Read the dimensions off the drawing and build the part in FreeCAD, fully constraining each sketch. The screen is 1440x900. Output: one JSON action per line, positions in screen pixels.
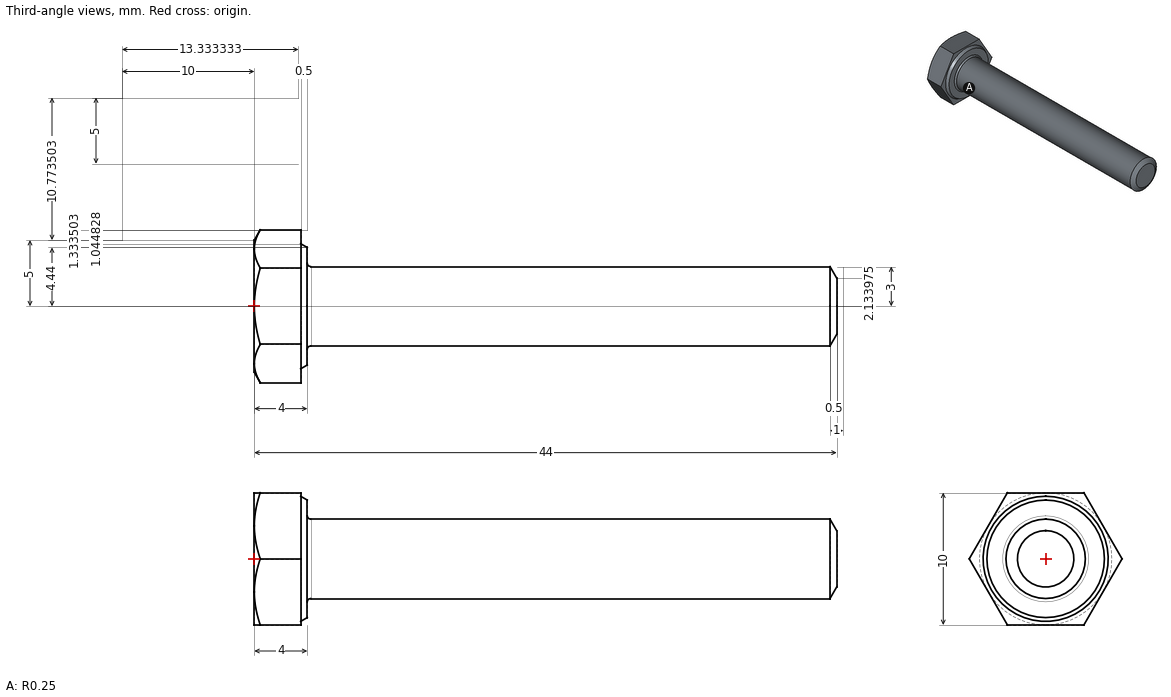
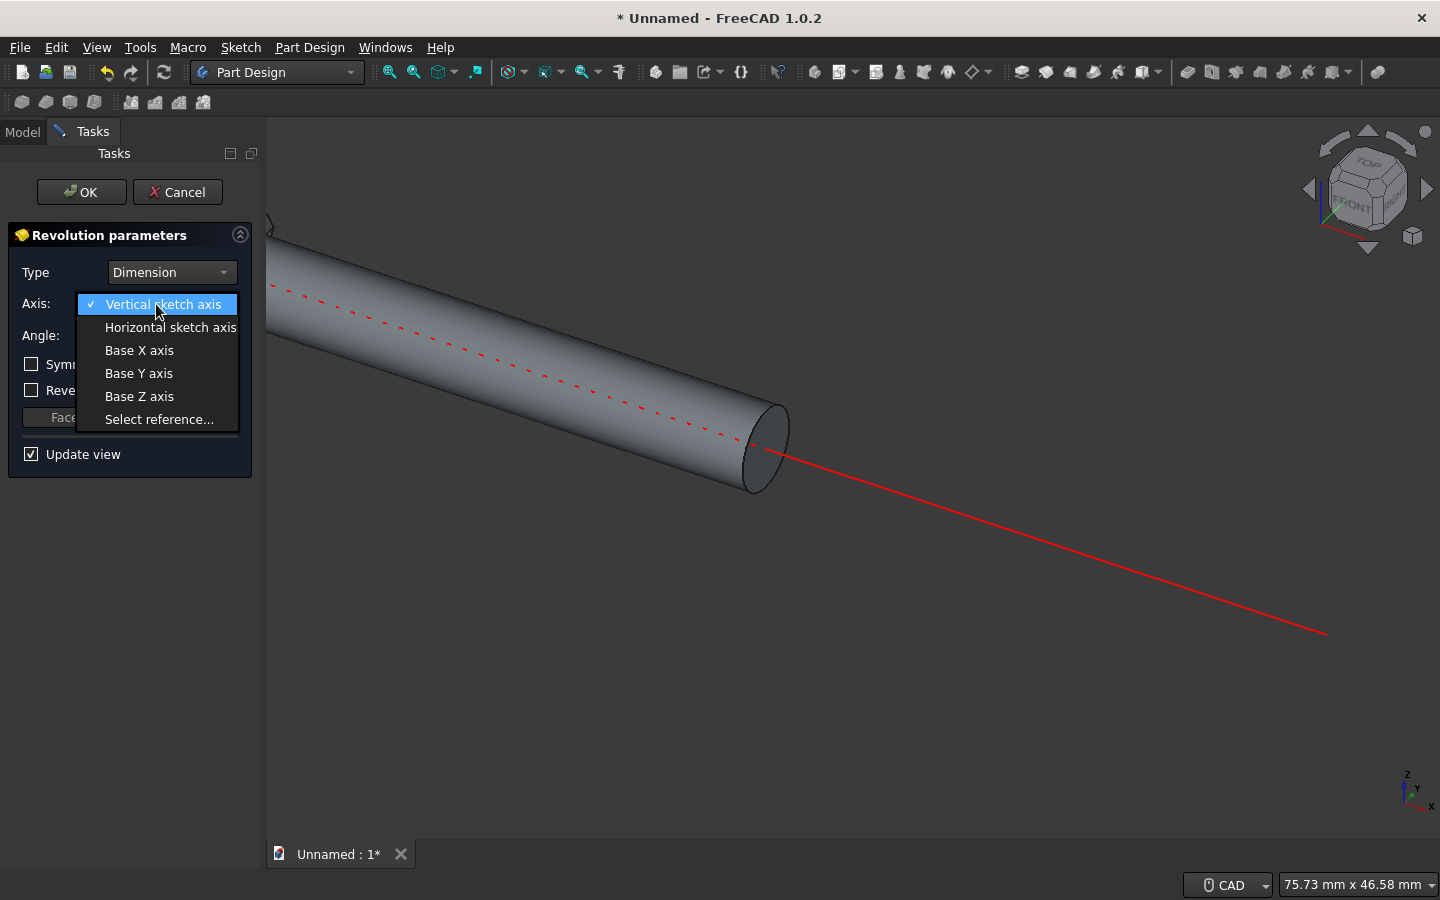
{"action": "left_click", "coordinate": [156, 328]}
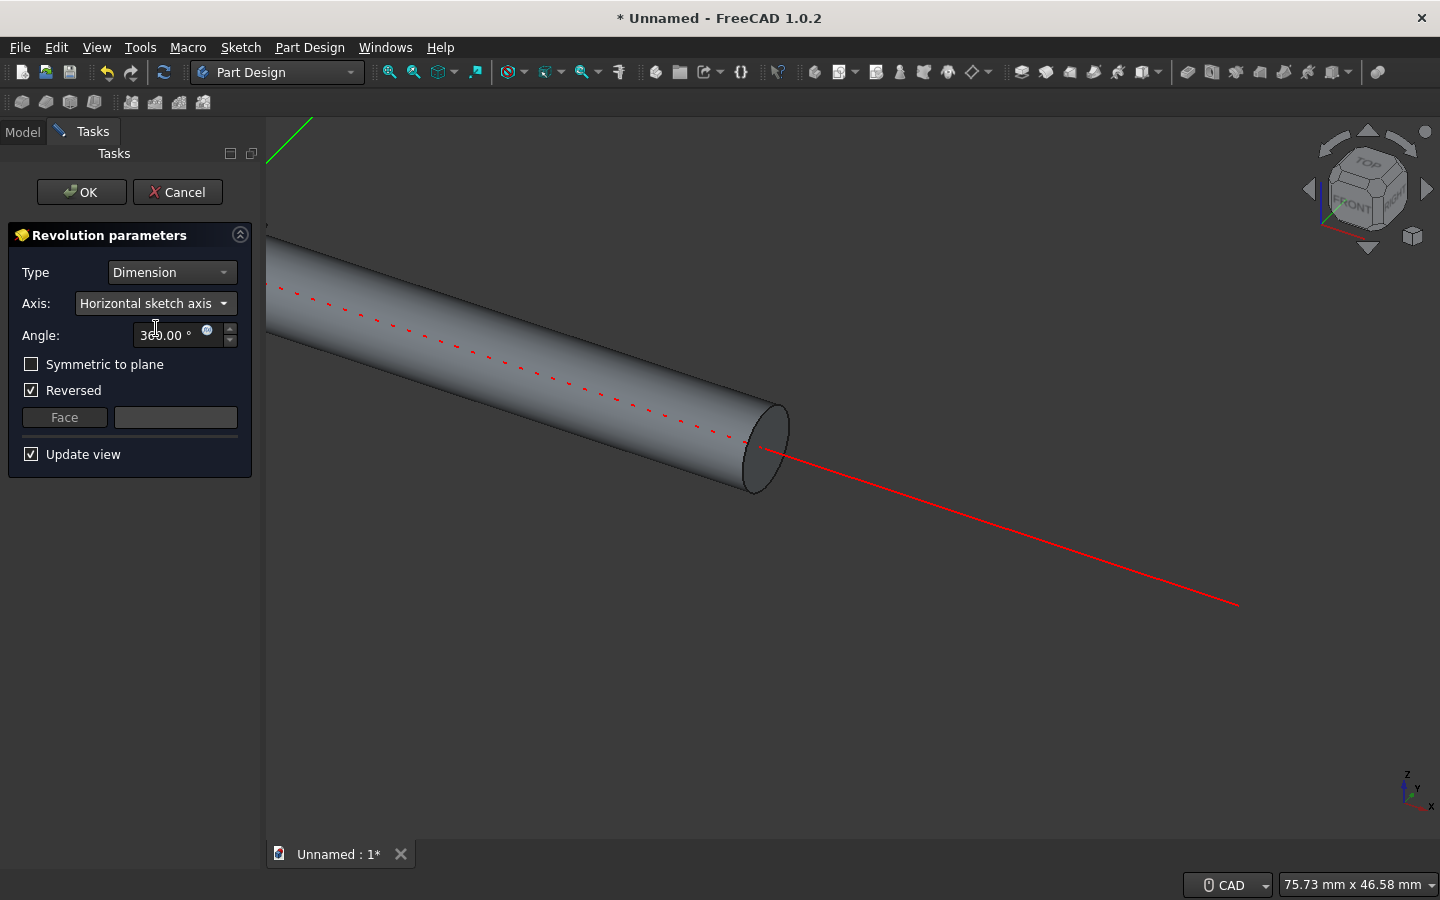
{"action": "left_click", "coordinate": [82, 192]}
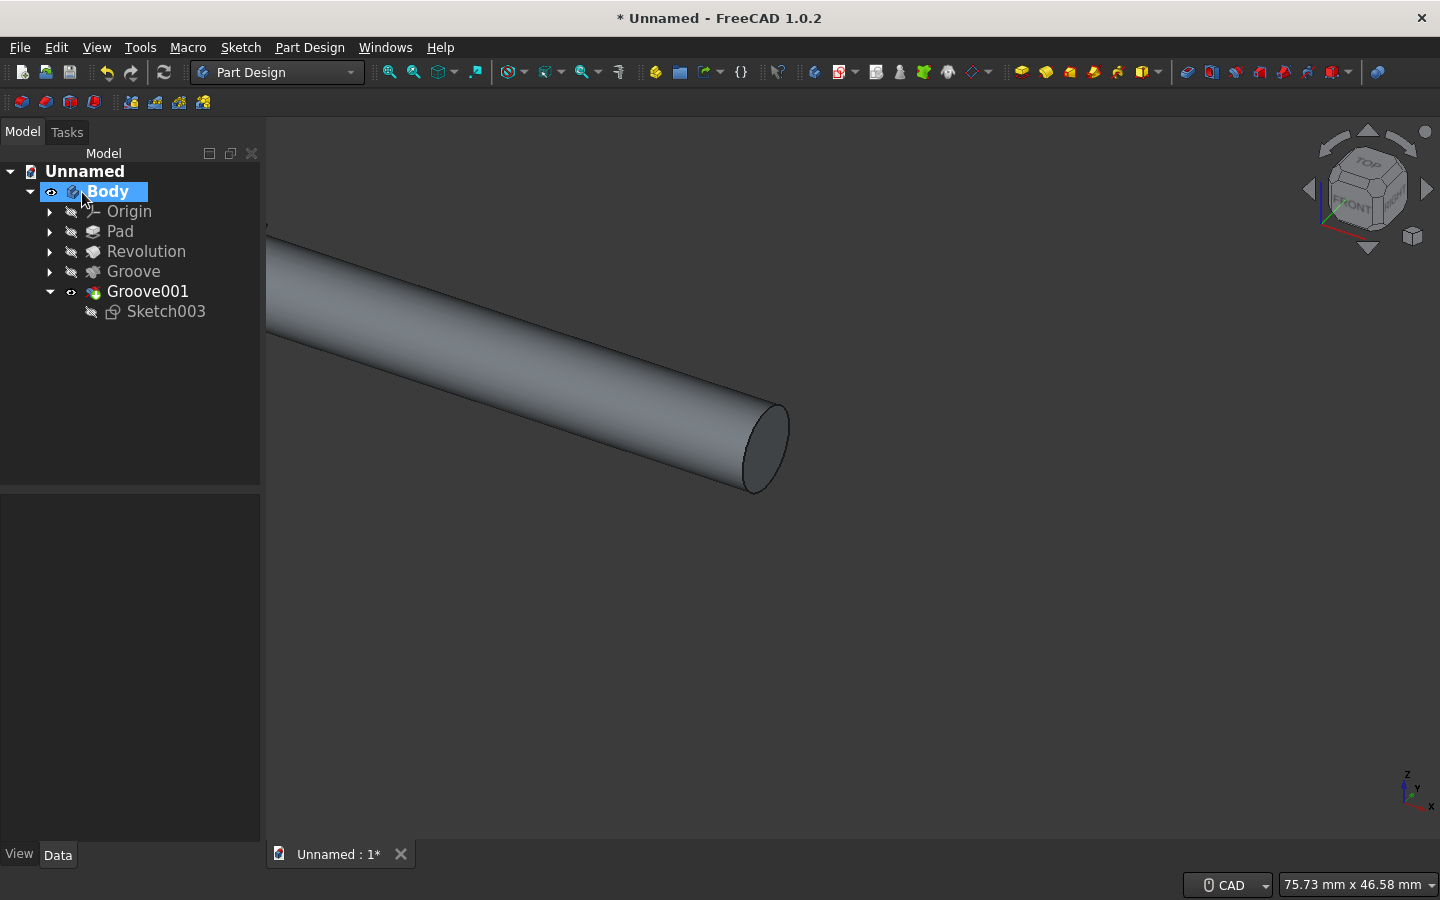
{"action": "left_click", "coordinate": [390, 72]}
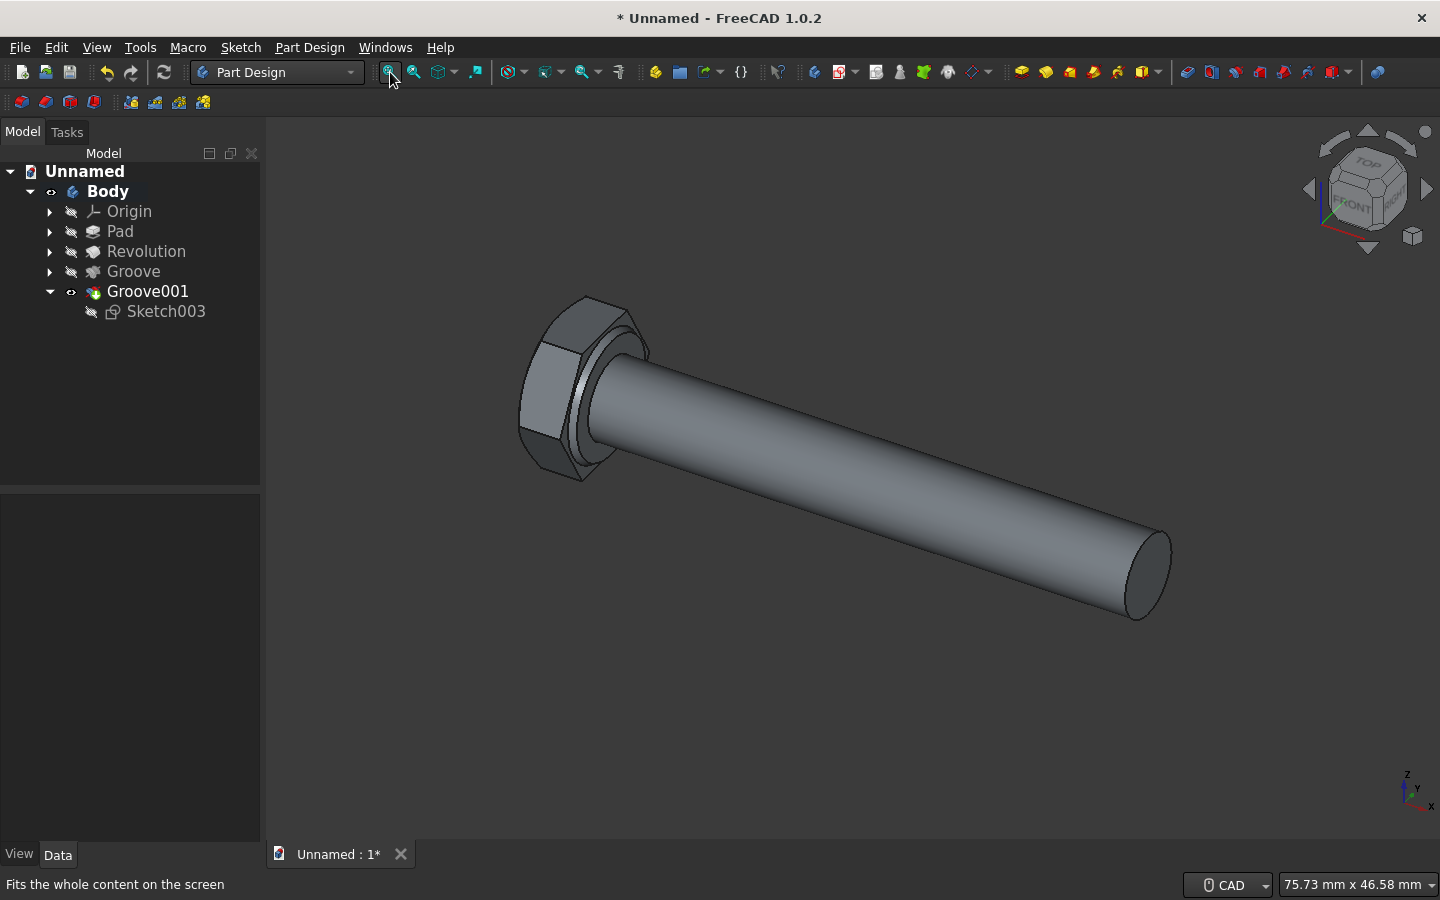
{"action": "key", "text": "0"}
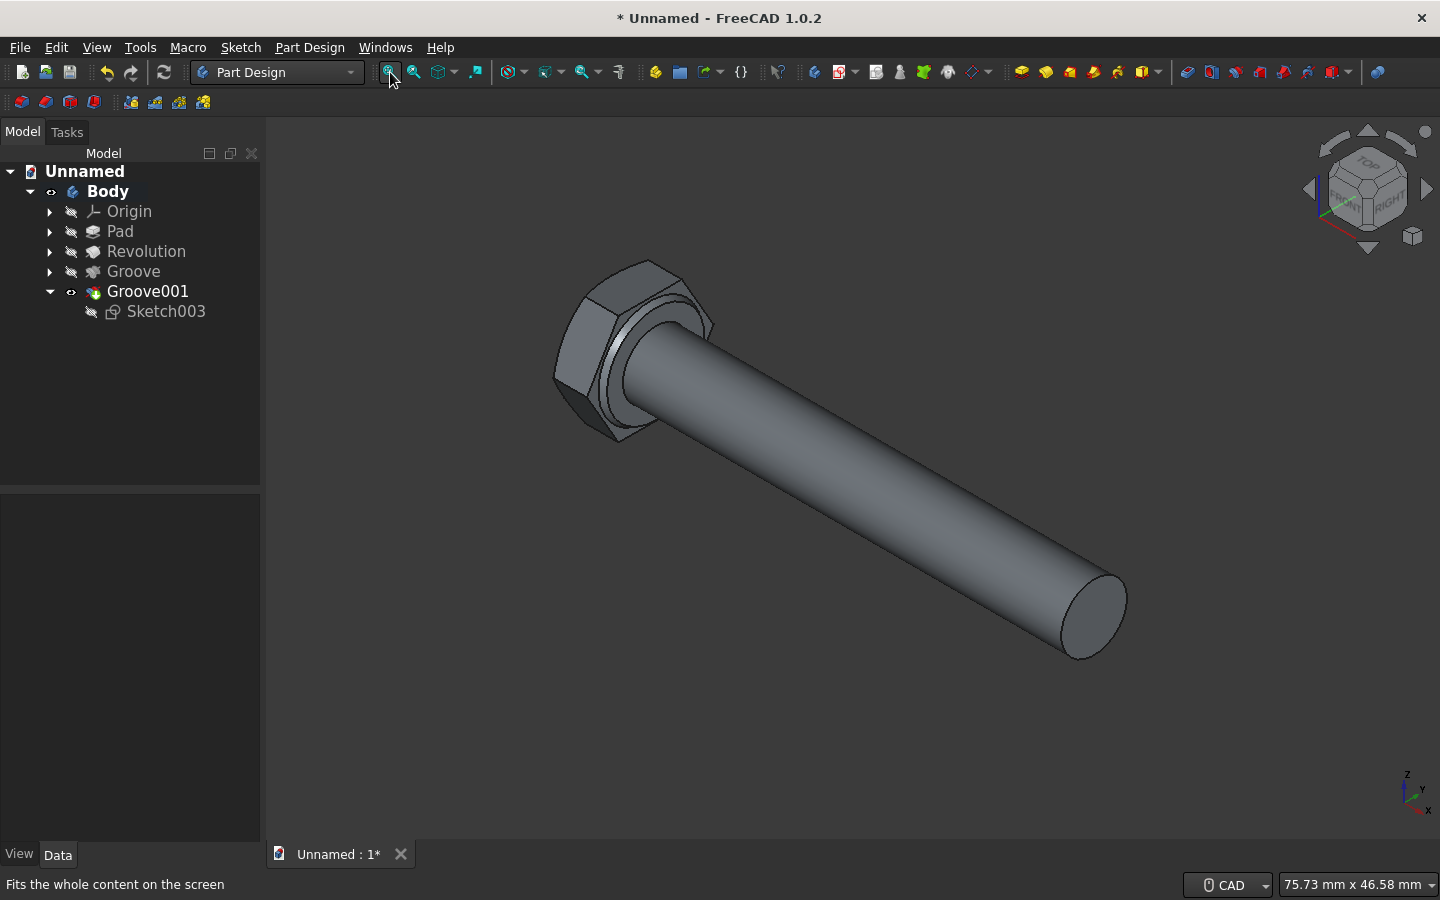
{"action": "key", "text": "2"}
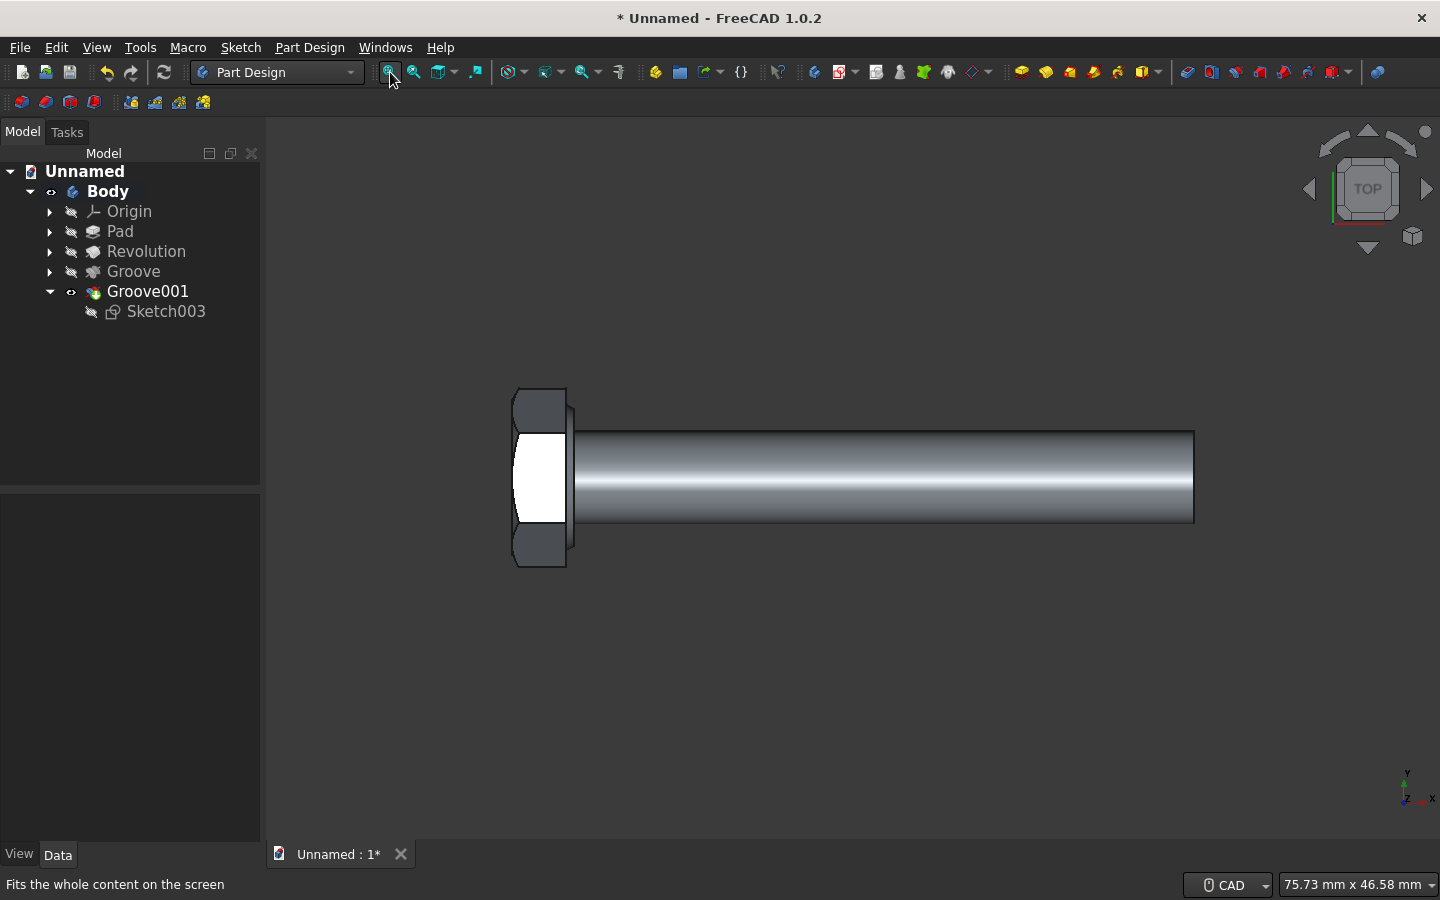
{"action": "key", "text": "1"}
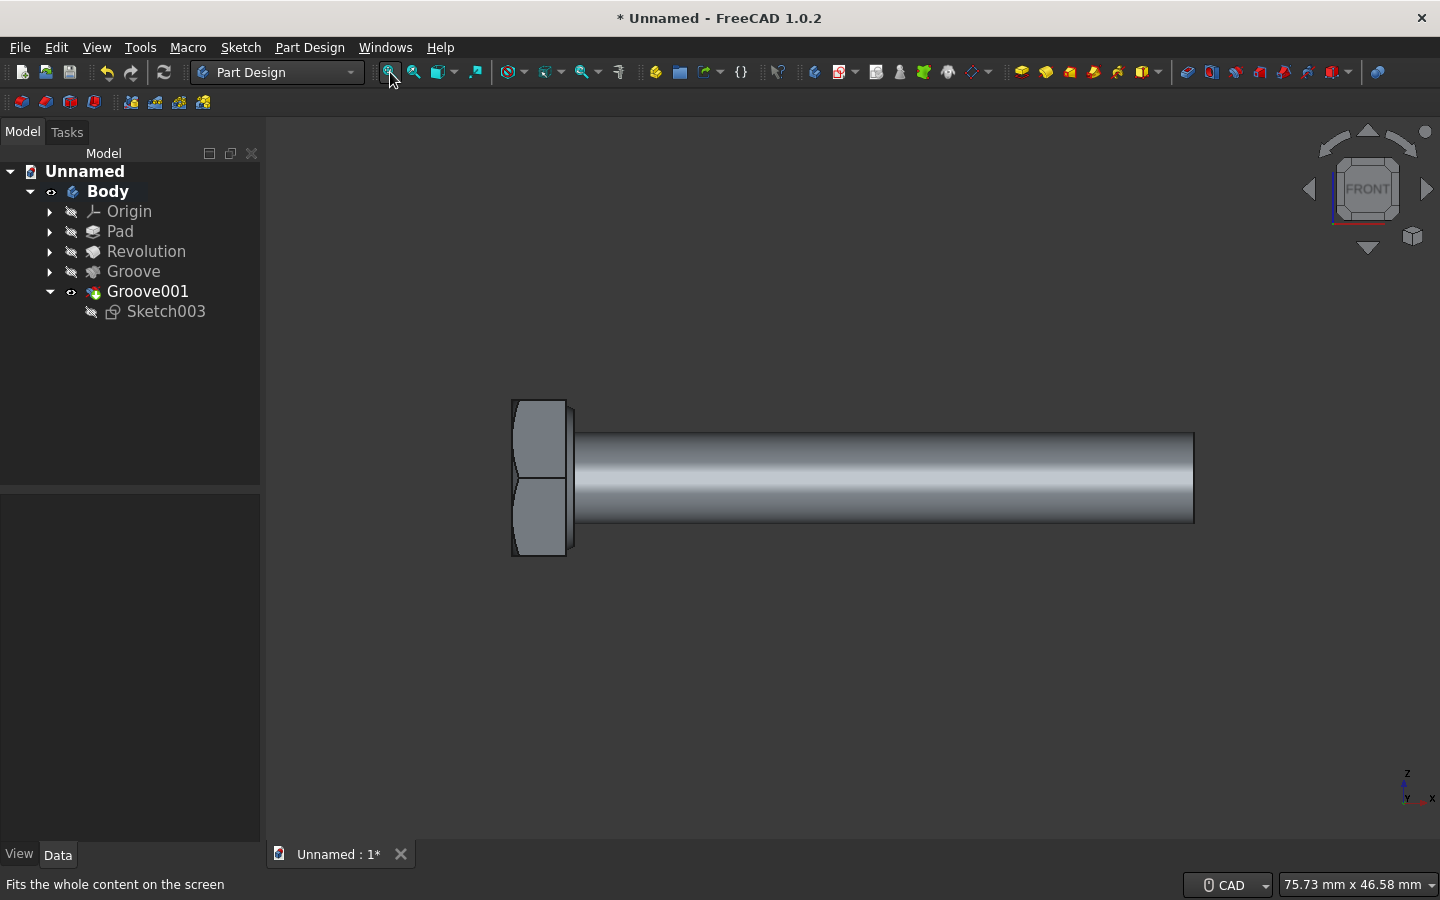
{"action": "key", "text": "3"}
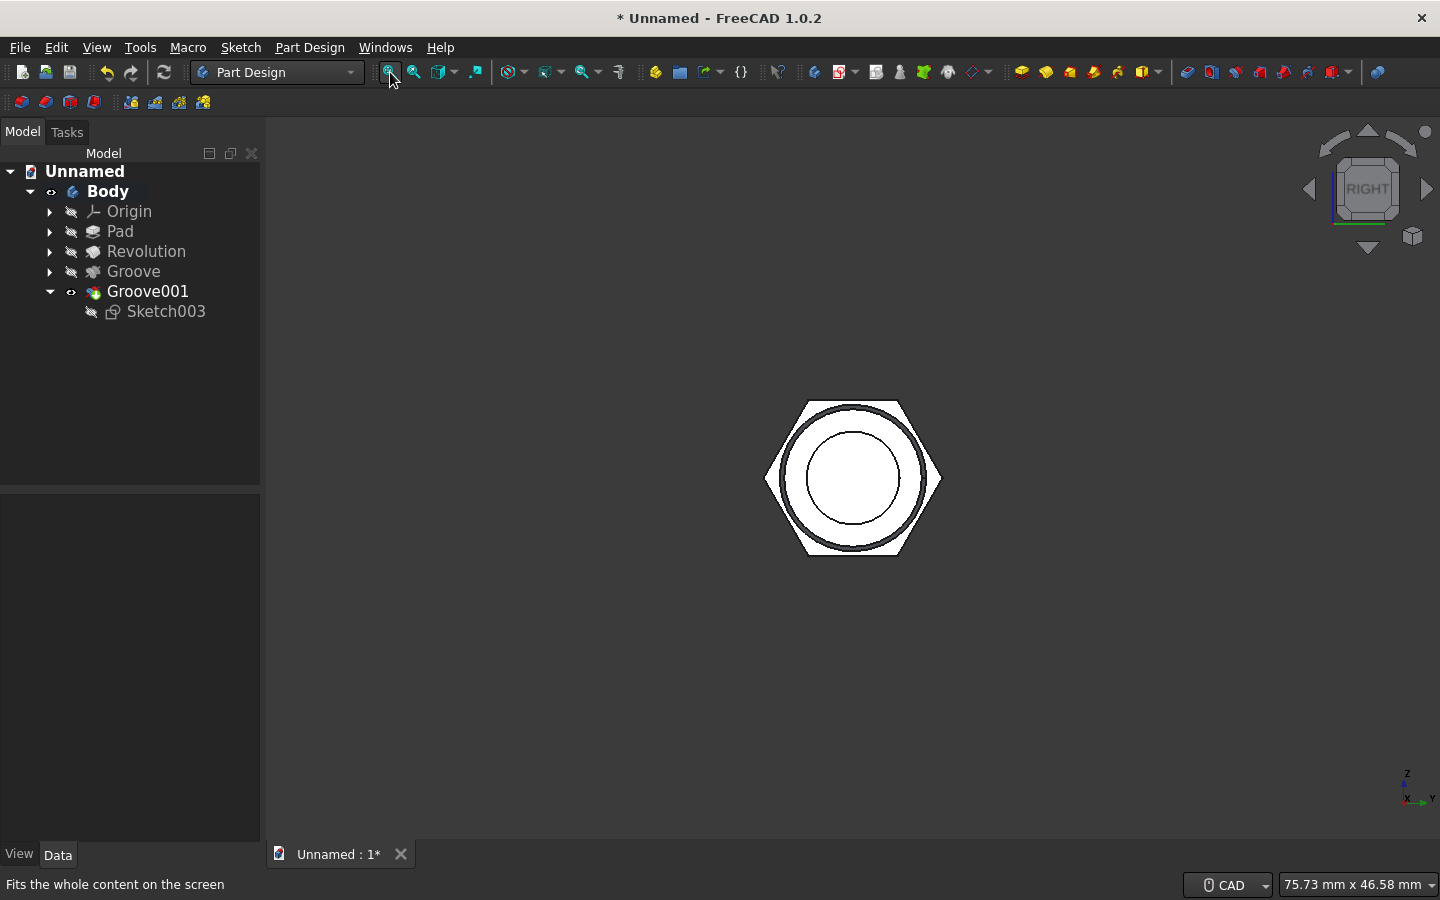
{"action": "left_click", "coordinate": [390, 72]}